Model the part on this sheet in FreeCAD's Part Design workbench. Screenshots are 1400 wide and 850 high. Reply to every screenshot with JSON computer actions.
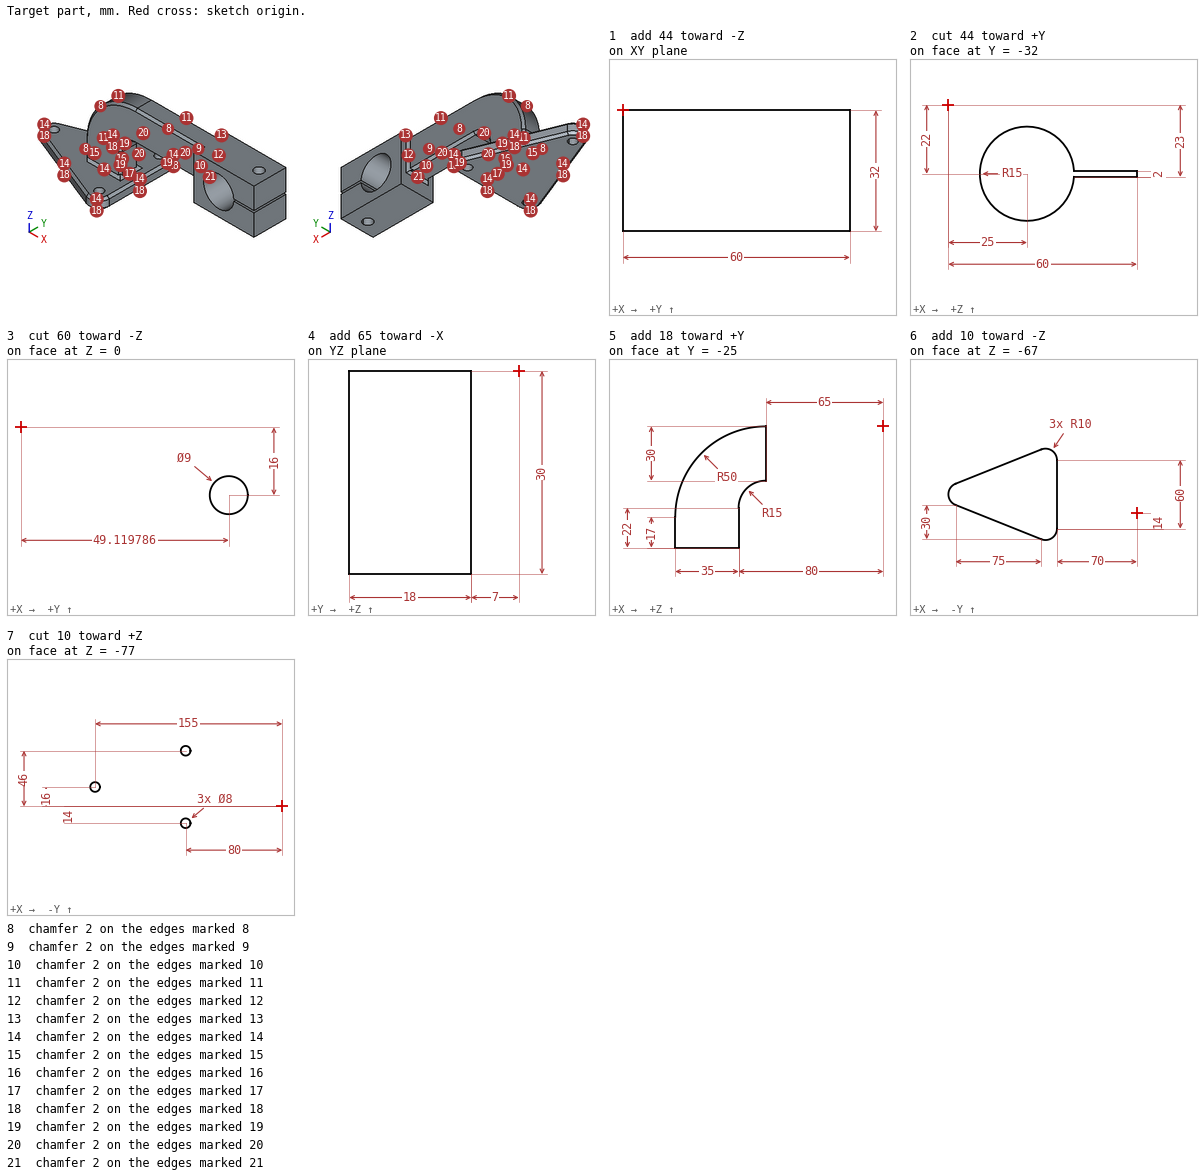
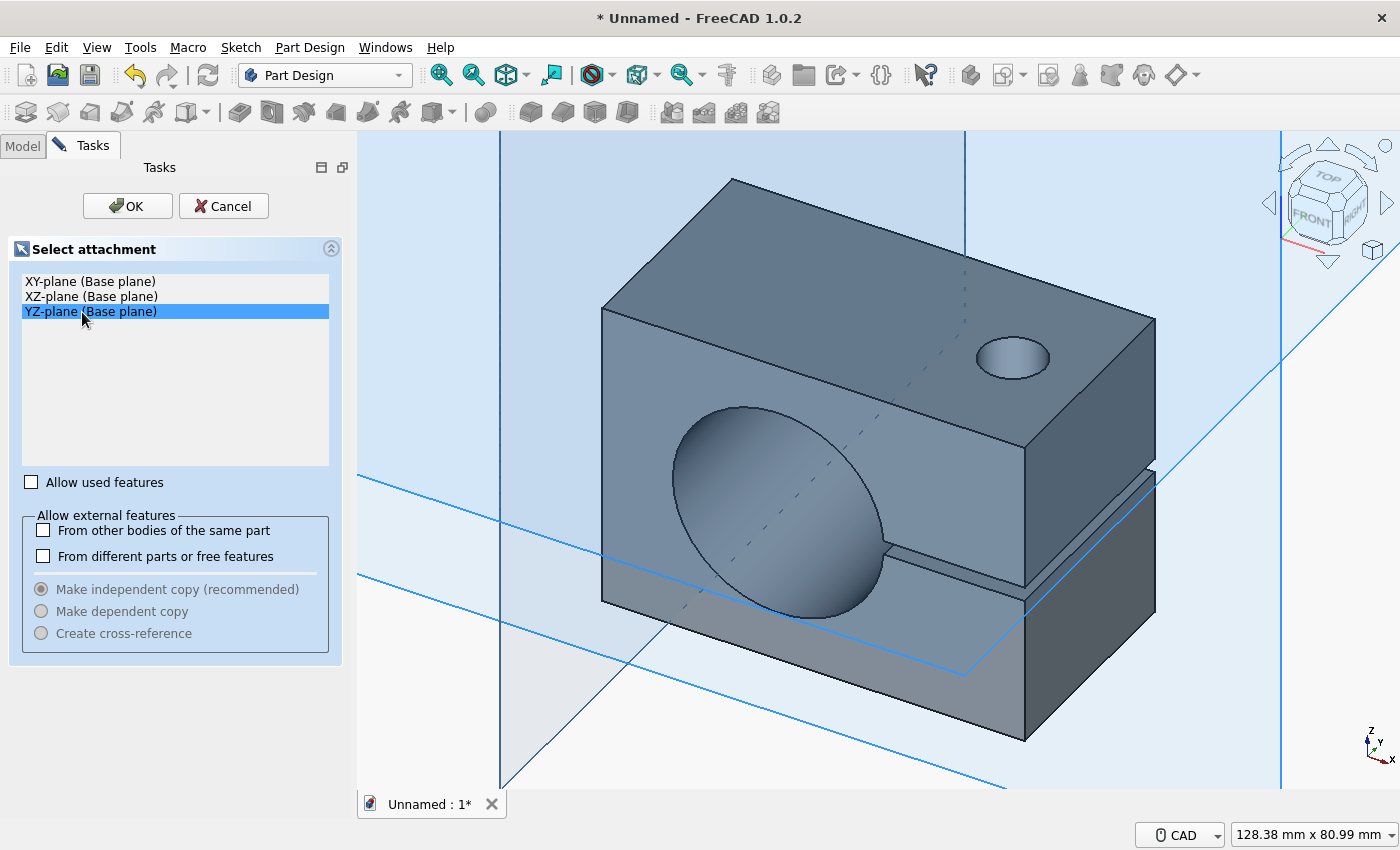
{"action": "left_click", "coordinate": [128, 206]}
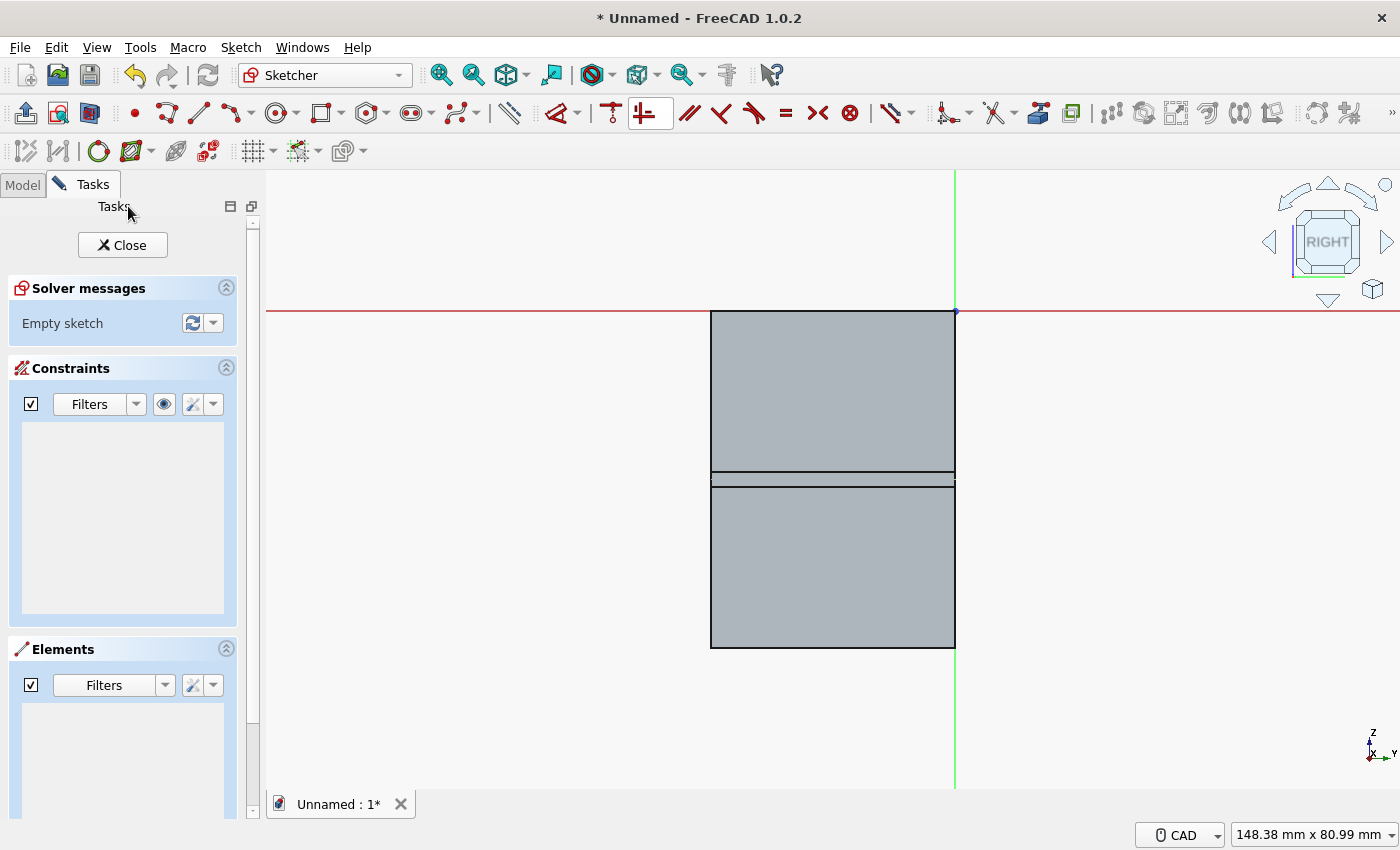
{"action": "left_click", "coordinate": [90, 114]}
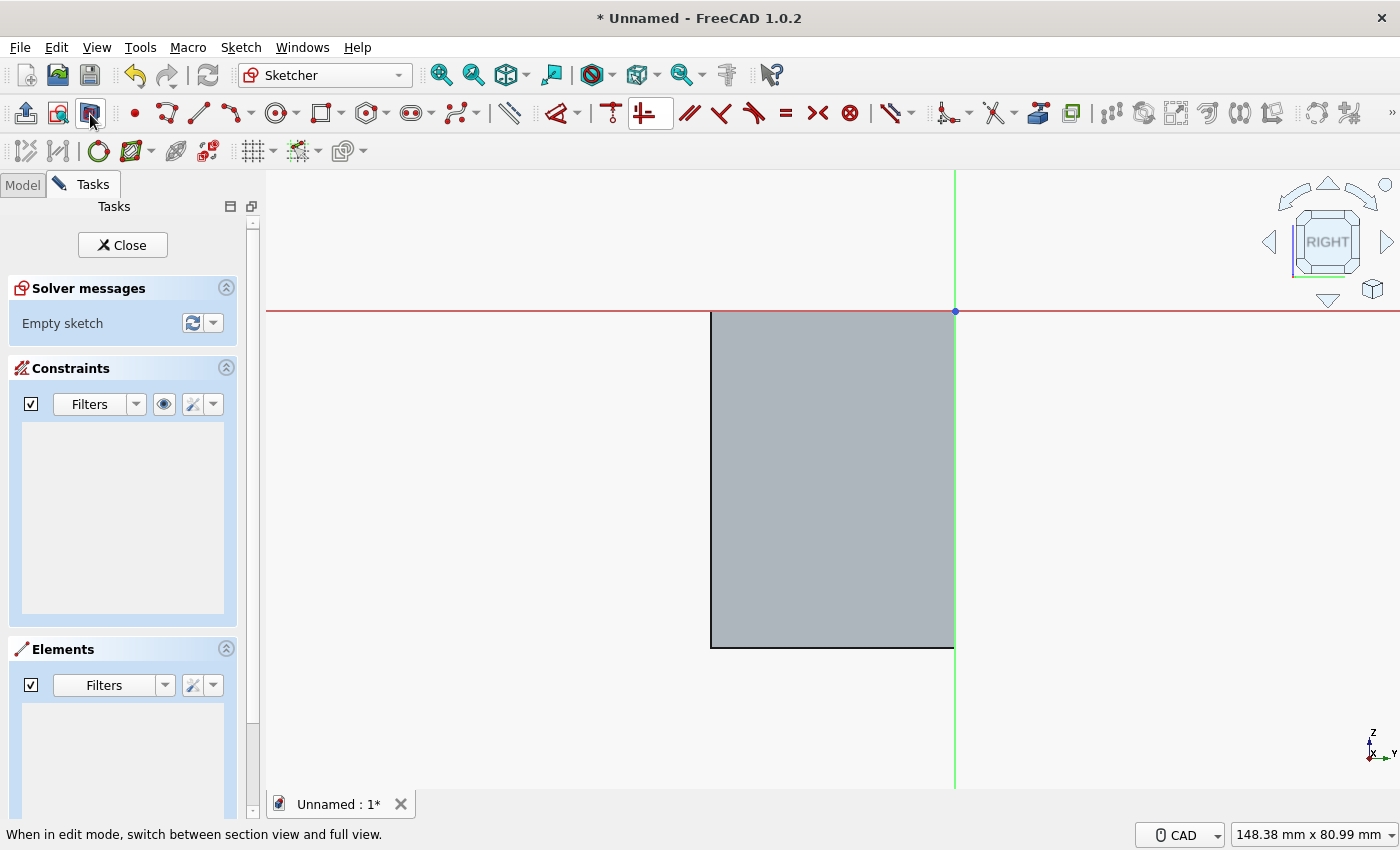
{"action": "scroll", "coordinate": [976, 361], "scroll_direction": "up", "scroll_amount": 3}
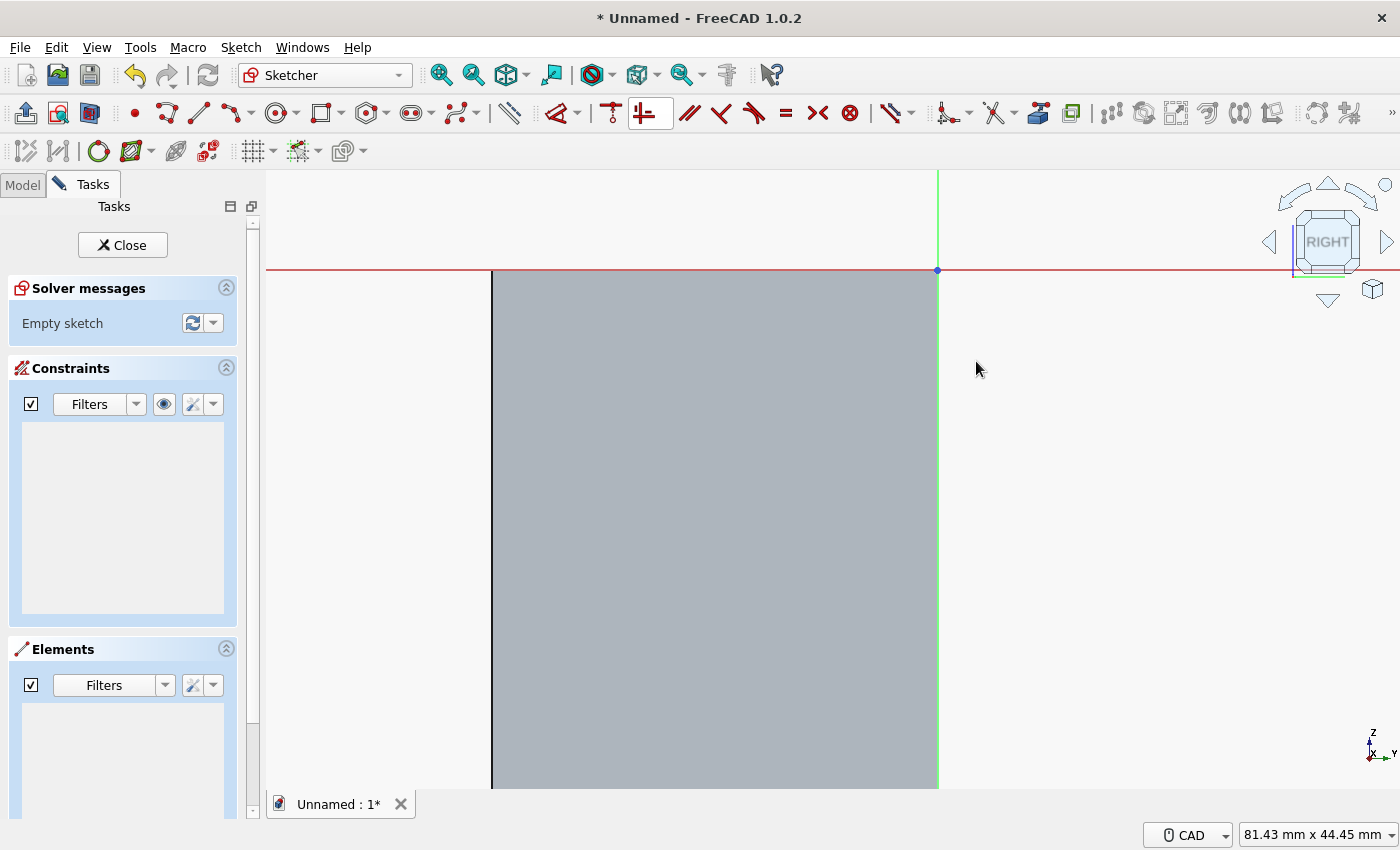
{"action": "left_click", "coordinate": [322, 114]}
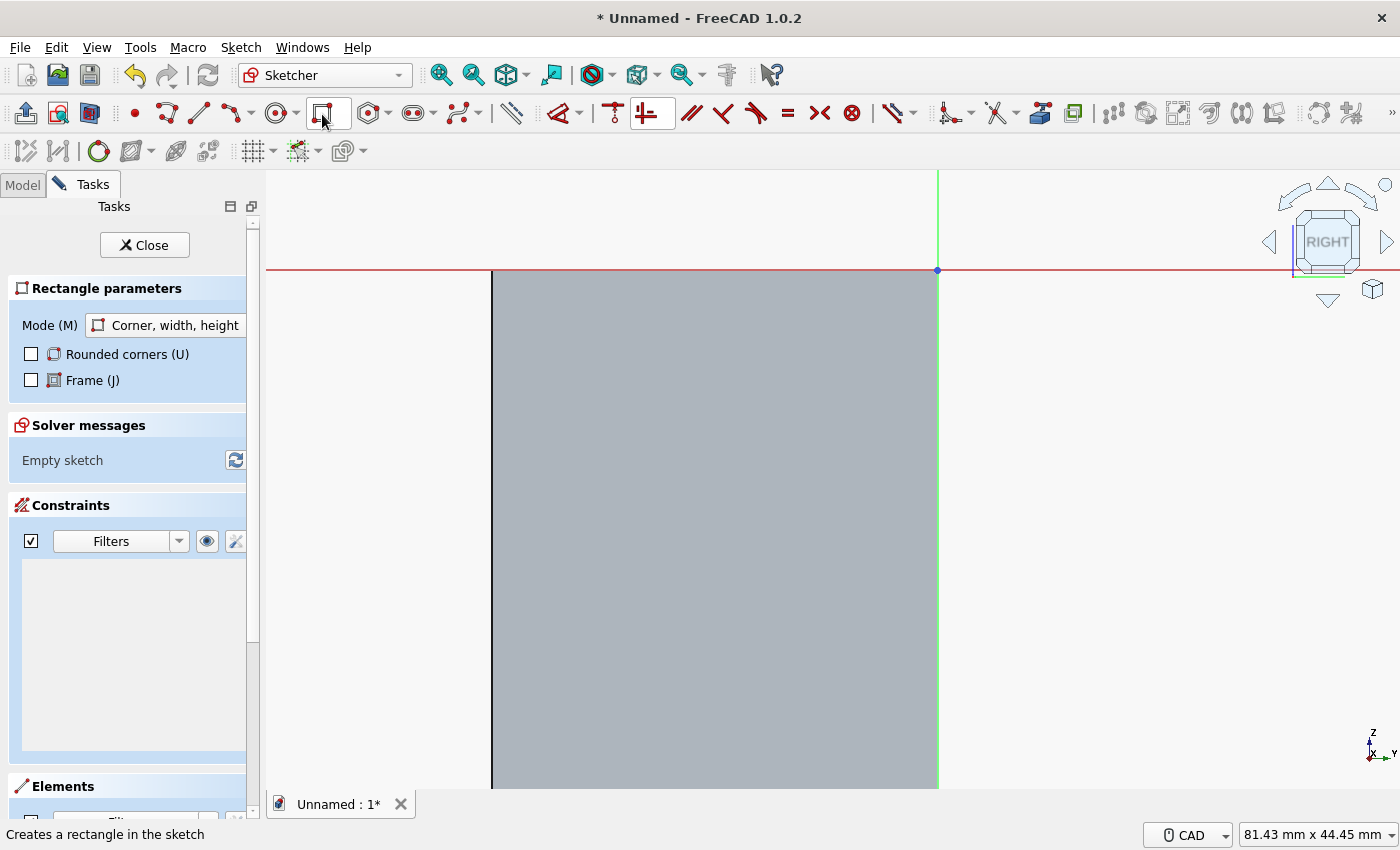
{"action": "left_click", "coordinate": [590, 270]}
{"action": "mouse_move", "coordinate": [840, 688]}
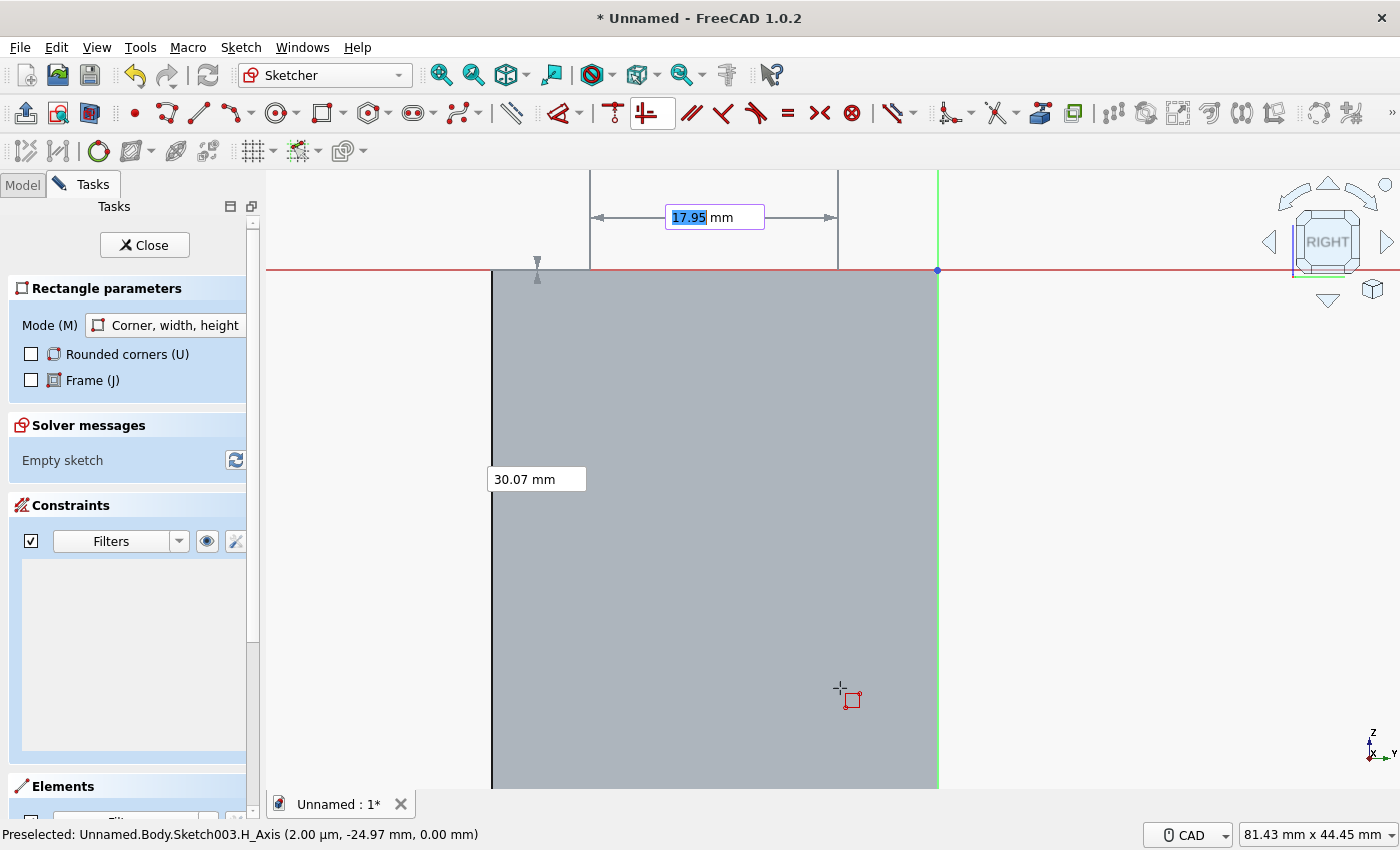
{"action": "type", "text": "18"}
{"action": "key", "text": "Tab"}
{"action": "type", "text": "30"}
{"action": "key", "text": "Return"}
{"action": "key", "text": "Escape"}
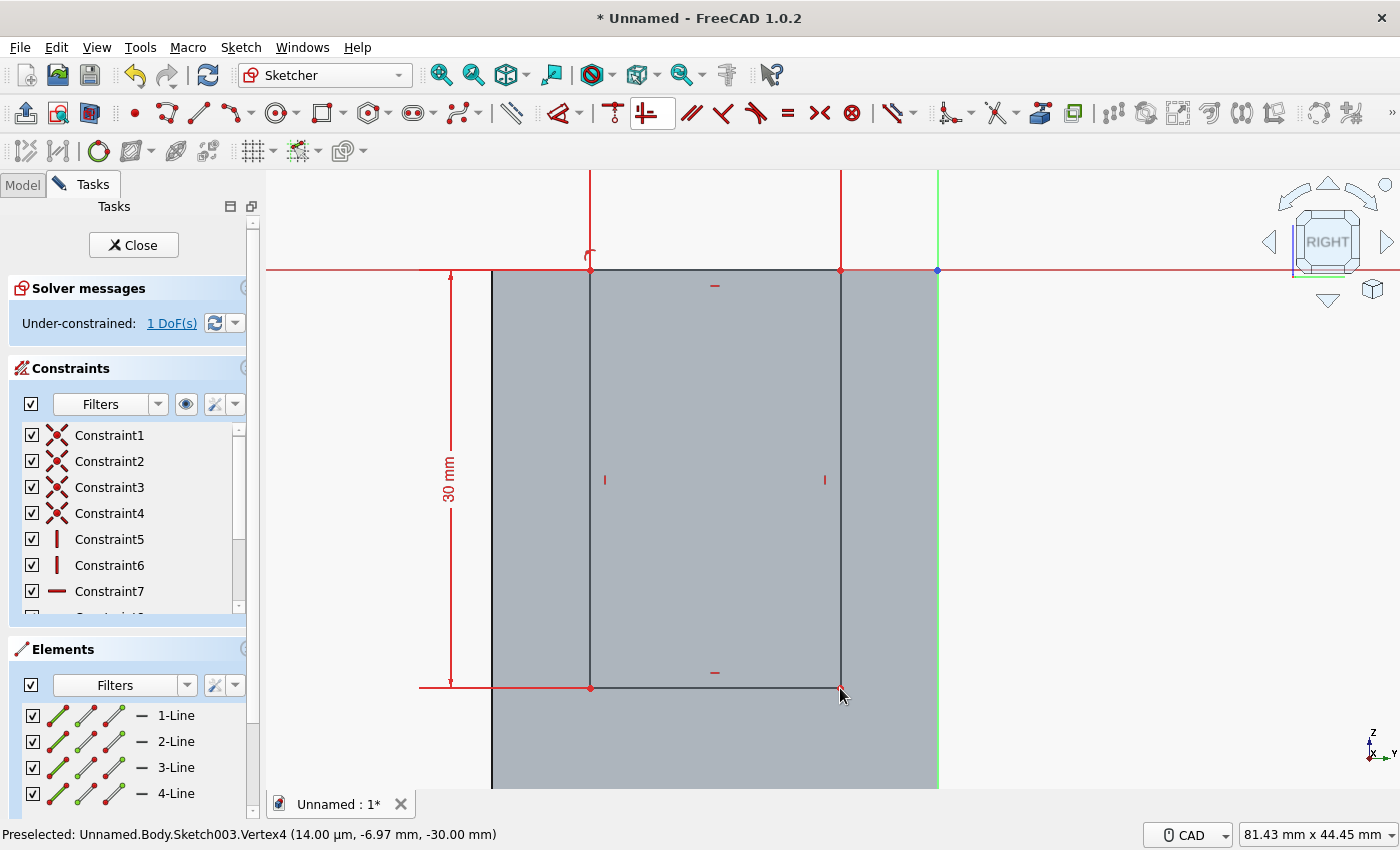
{"action": "left_click", "coordinate": [558, 114]}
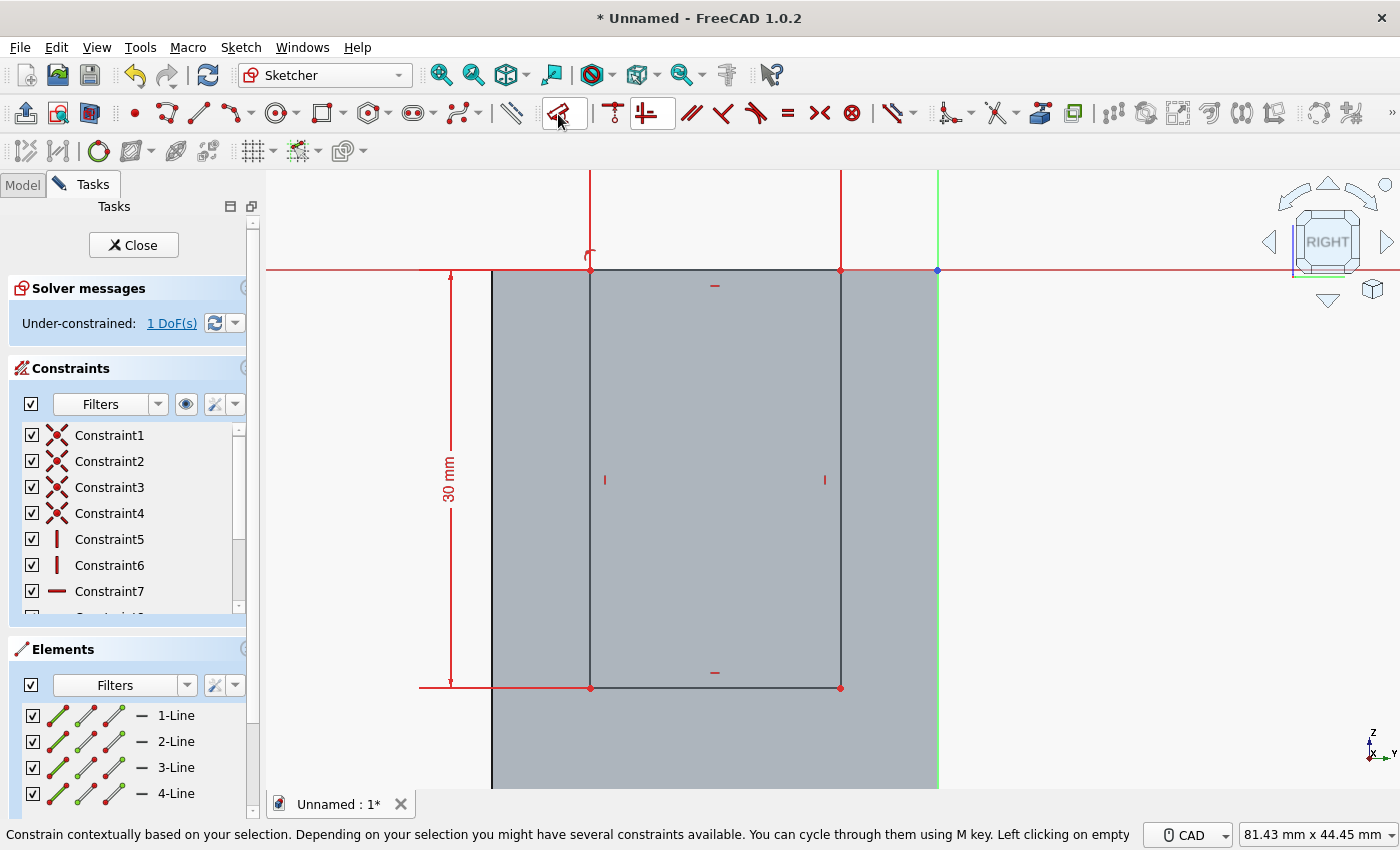
{"action": "left_click", "coordinate": [841, 688]}
{"action": "left_click", "coordinate": [889, 722]}